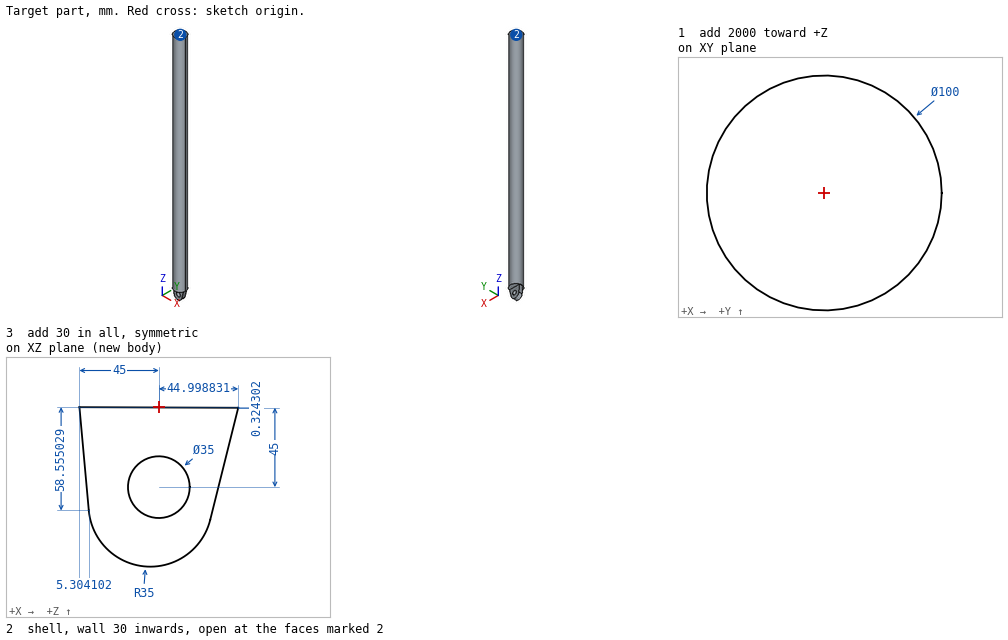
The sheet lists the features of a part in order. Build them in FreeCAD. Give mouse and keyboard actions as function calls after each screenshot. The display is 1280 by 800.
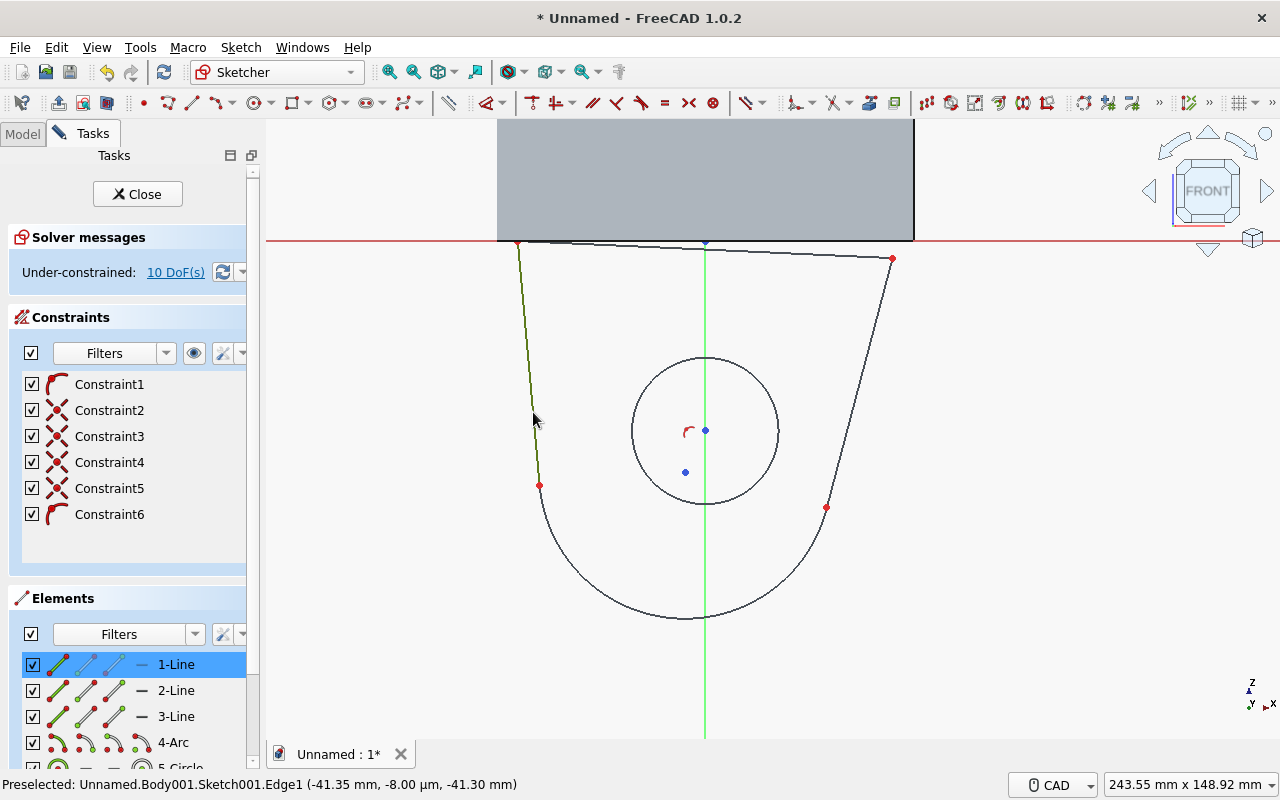
click(598, 590)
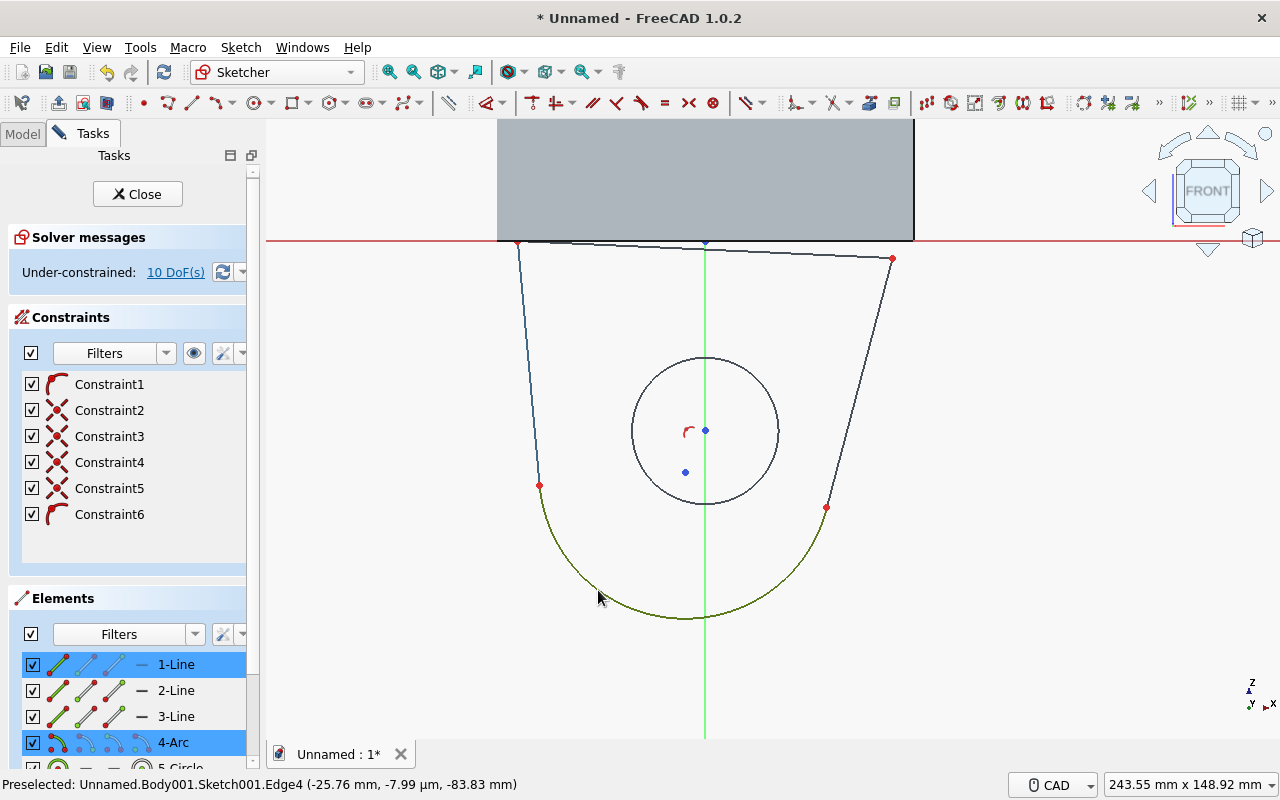
click(642, 104)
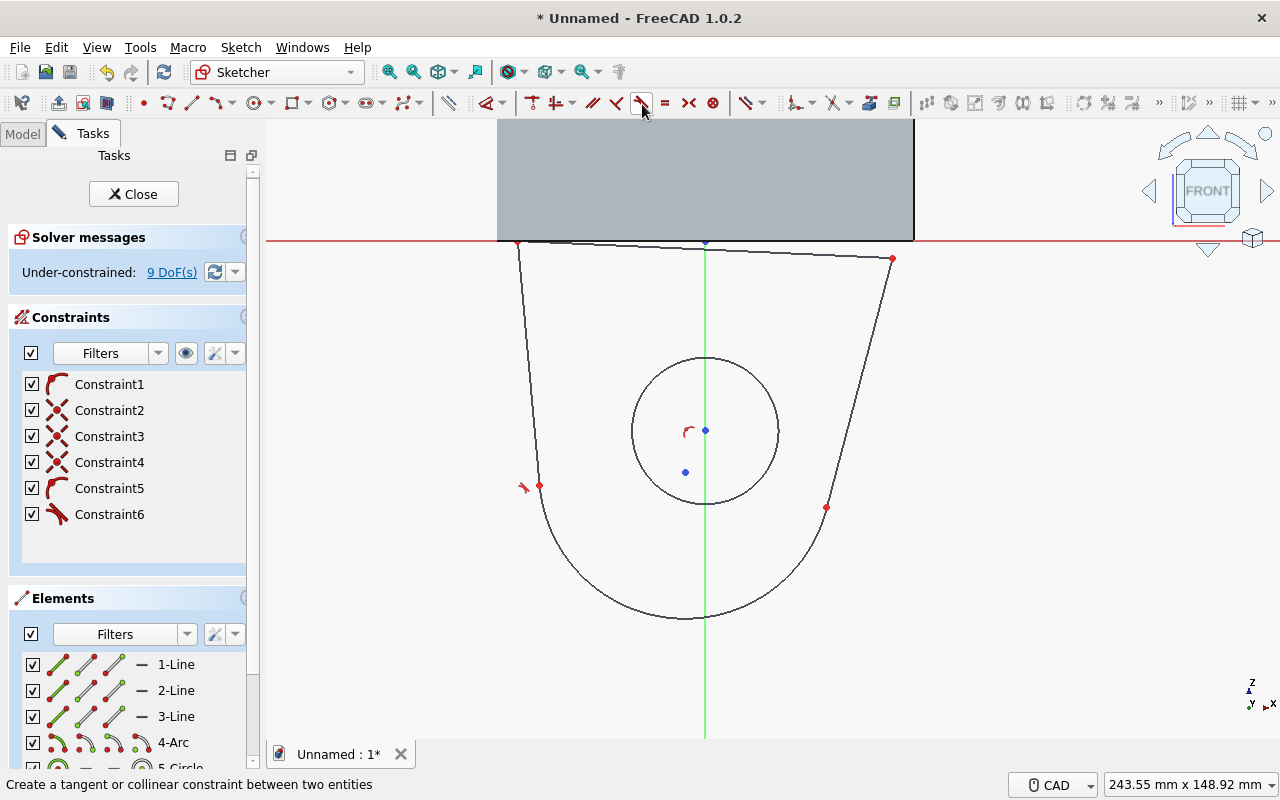
click(873, 333)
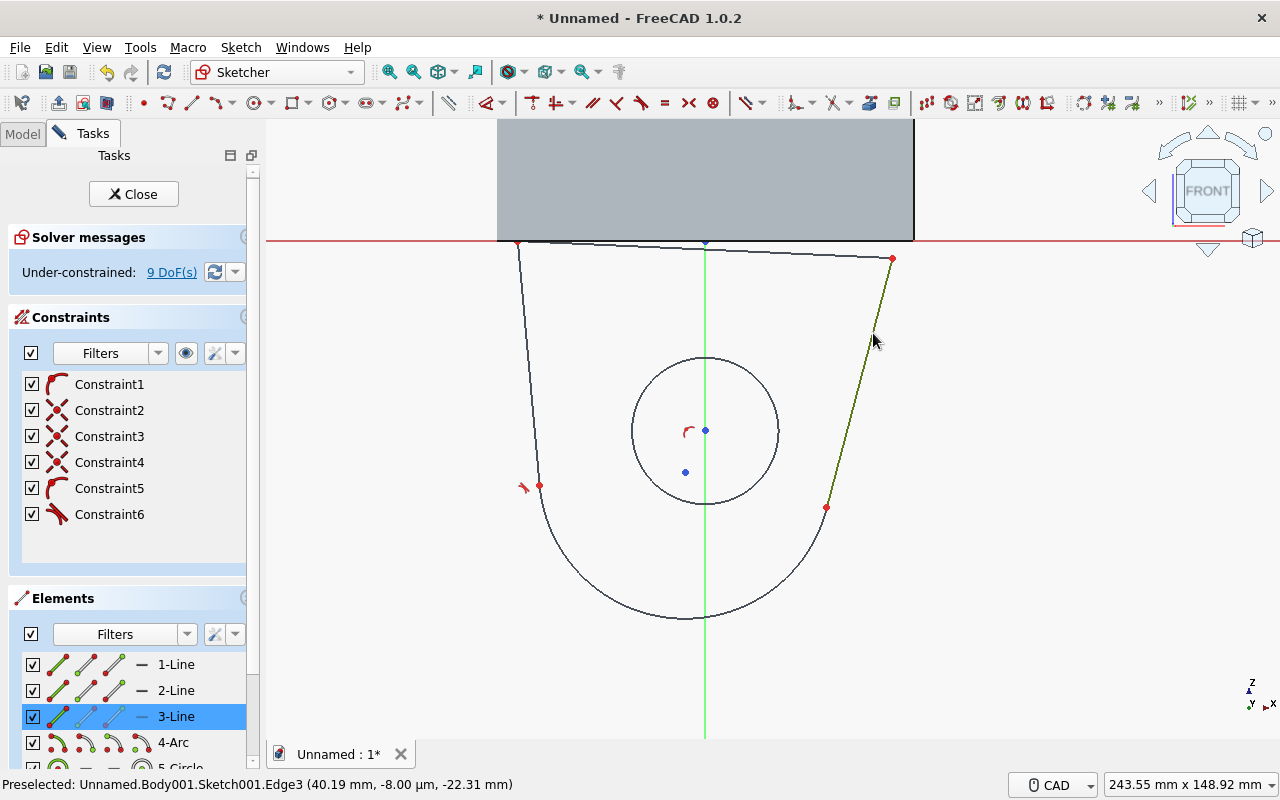
click(598, 590)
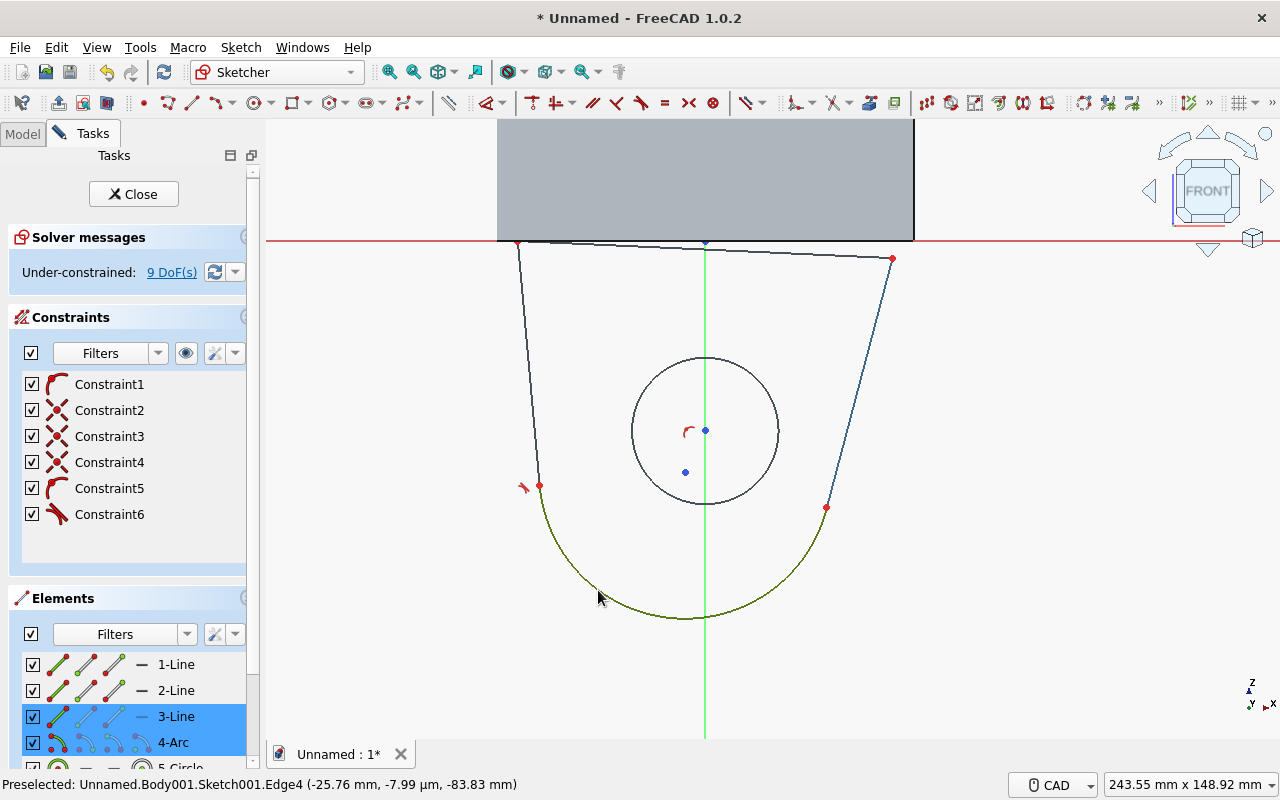
click(642, 104)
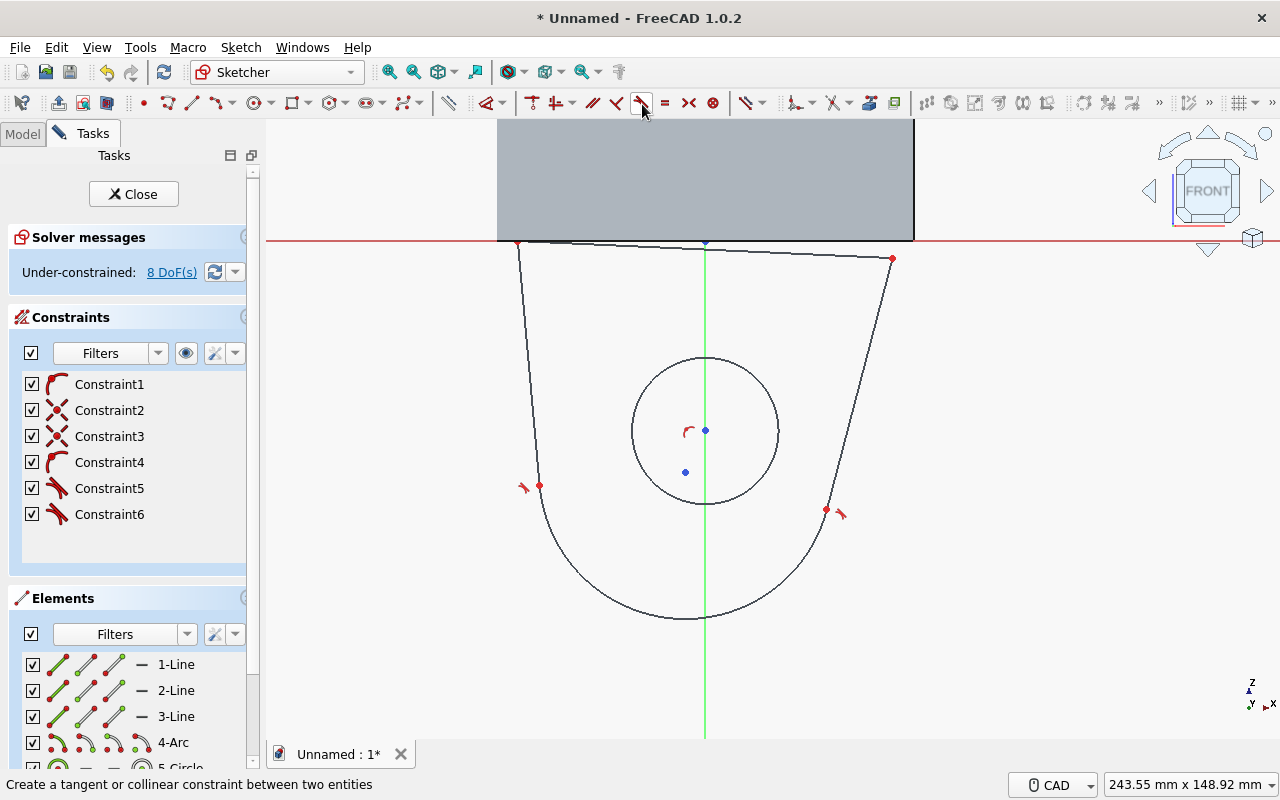
key(d)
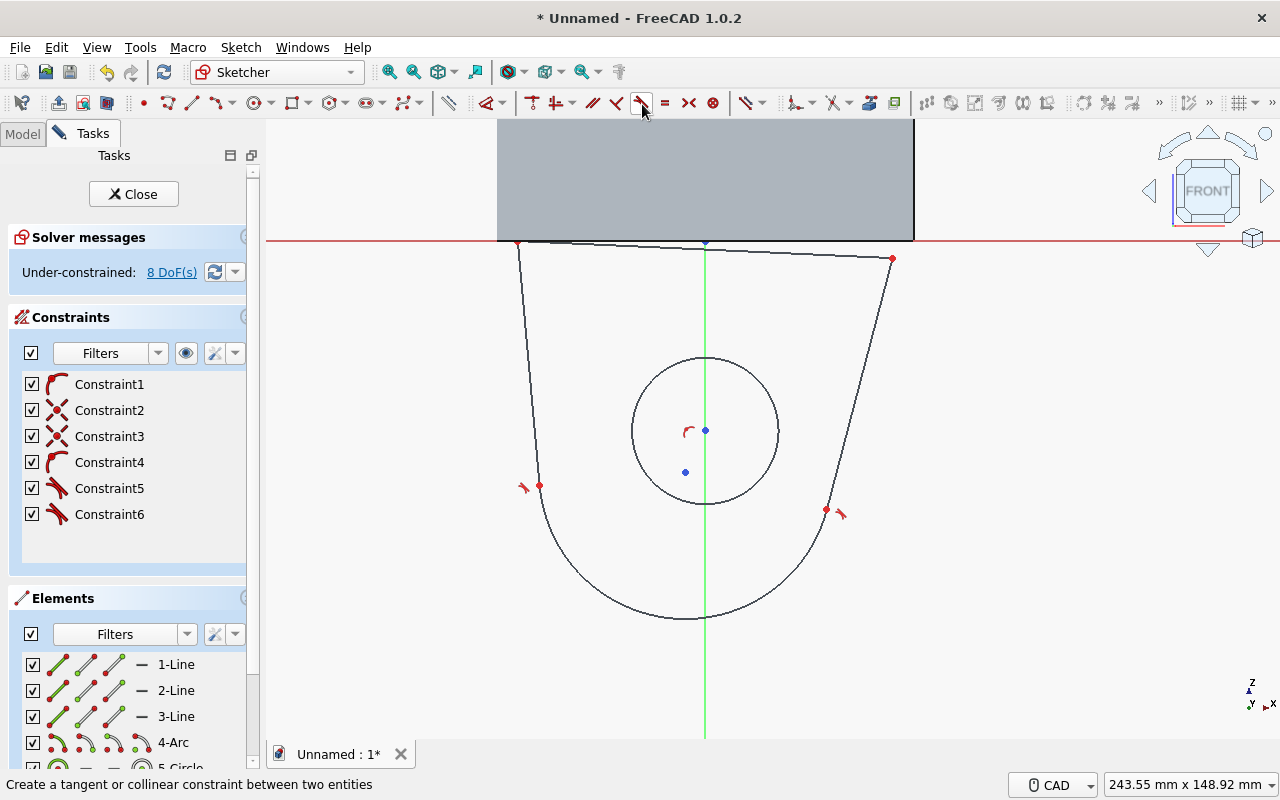
click(598, 590)
click(579, 616)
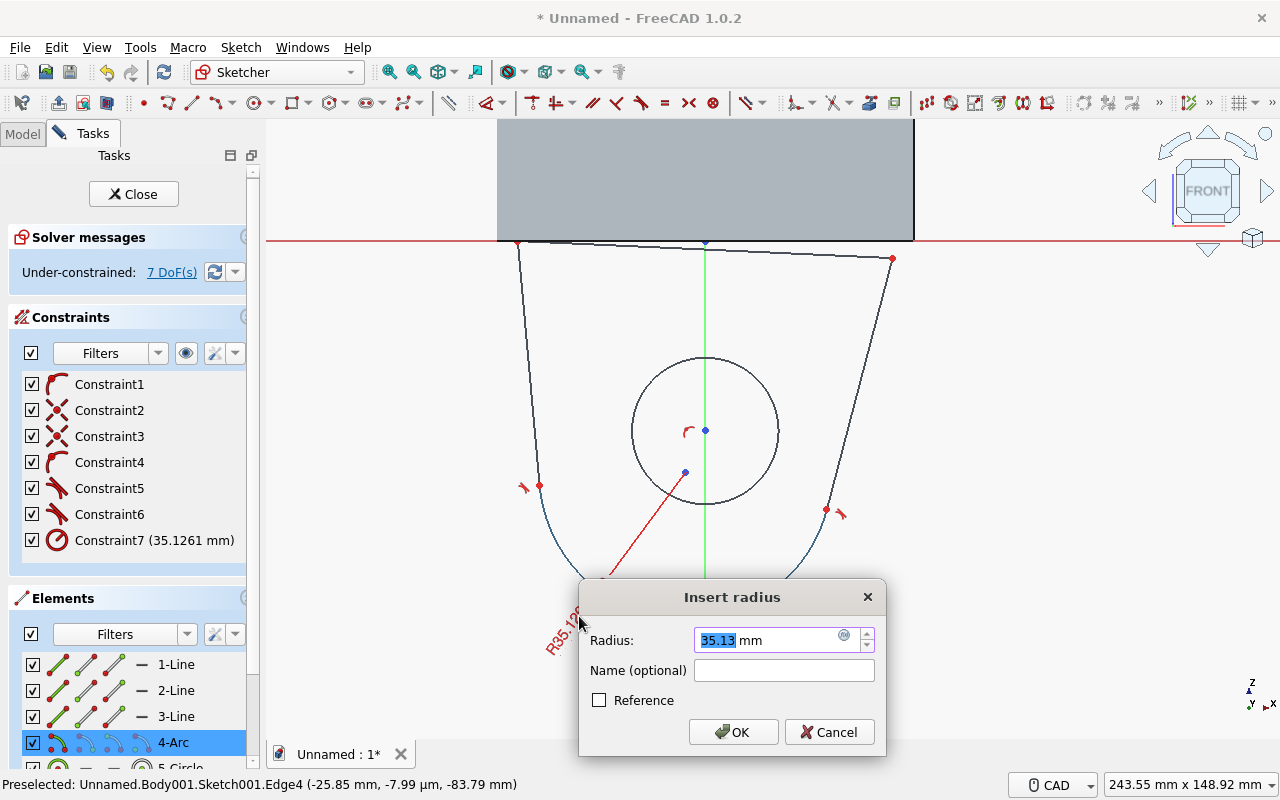
text(35)
key(Return)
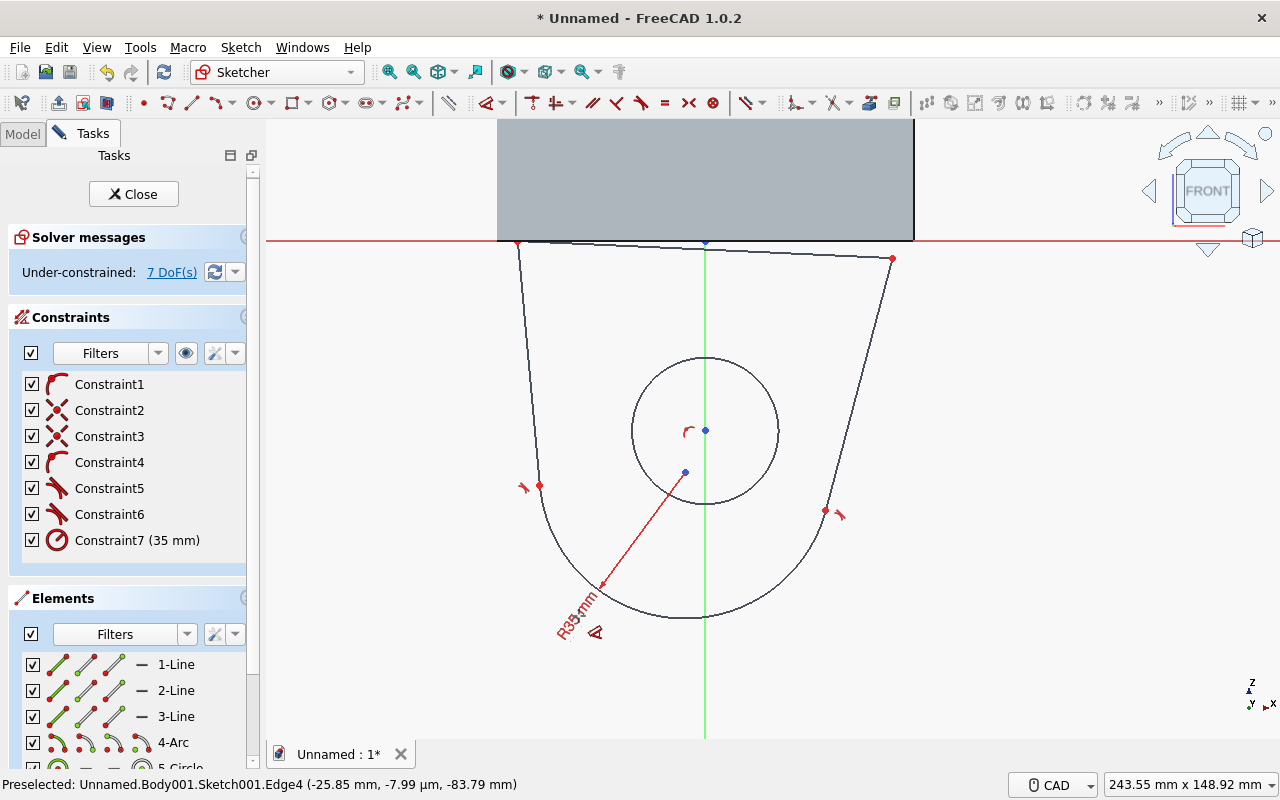
click(757, 379)
click(780, 356)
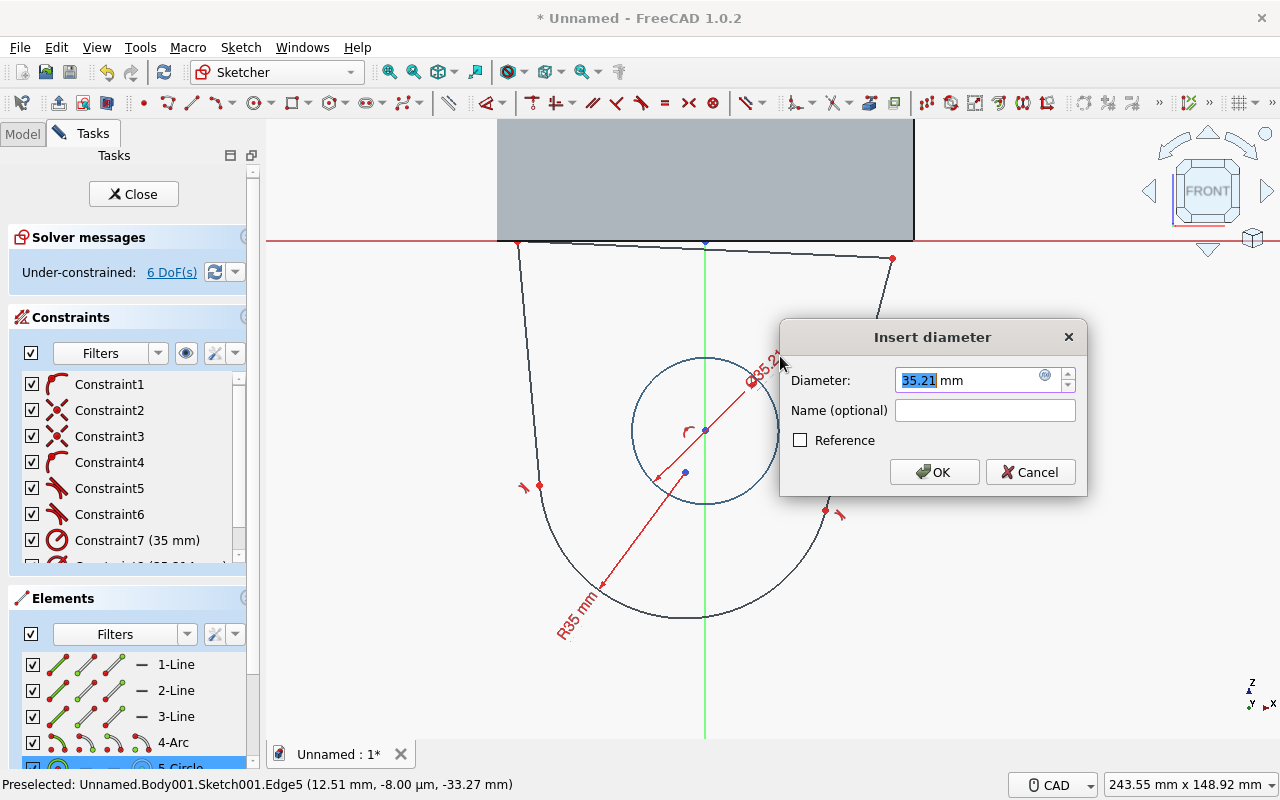
text(35)
key(Return)